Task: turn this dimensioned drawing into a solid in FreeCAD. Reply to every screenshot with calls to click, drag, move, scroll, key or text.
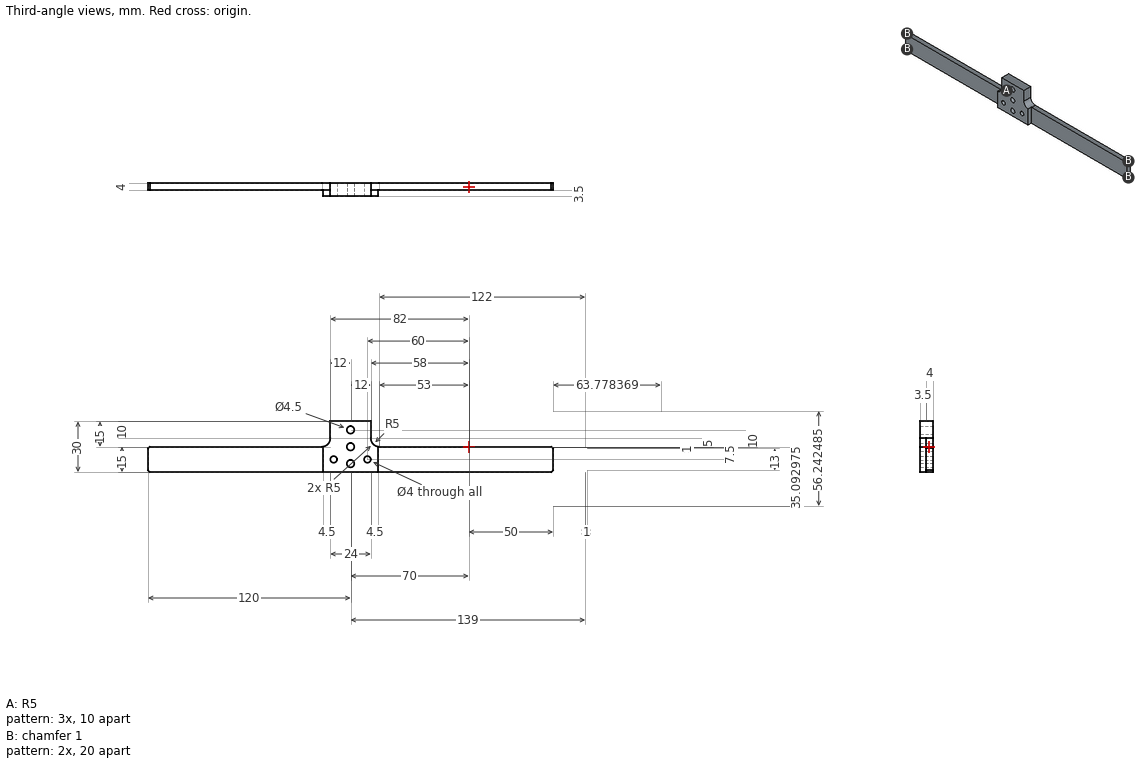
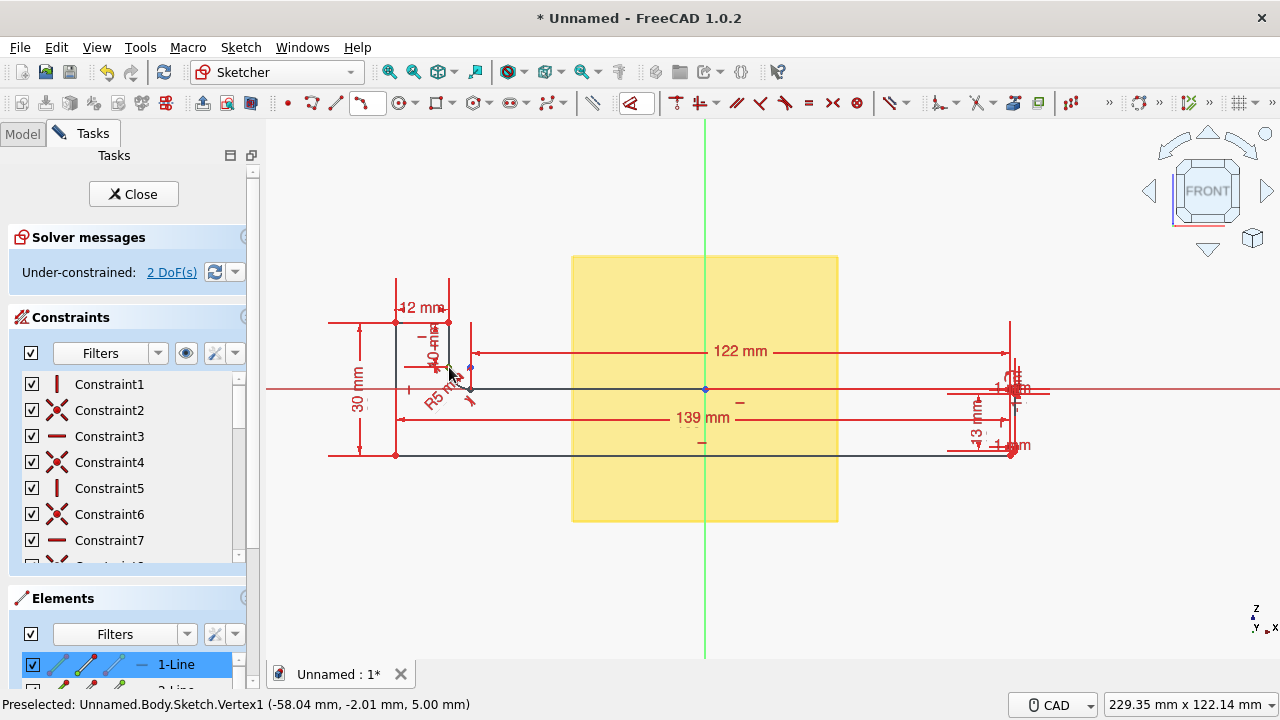
click(648, 104)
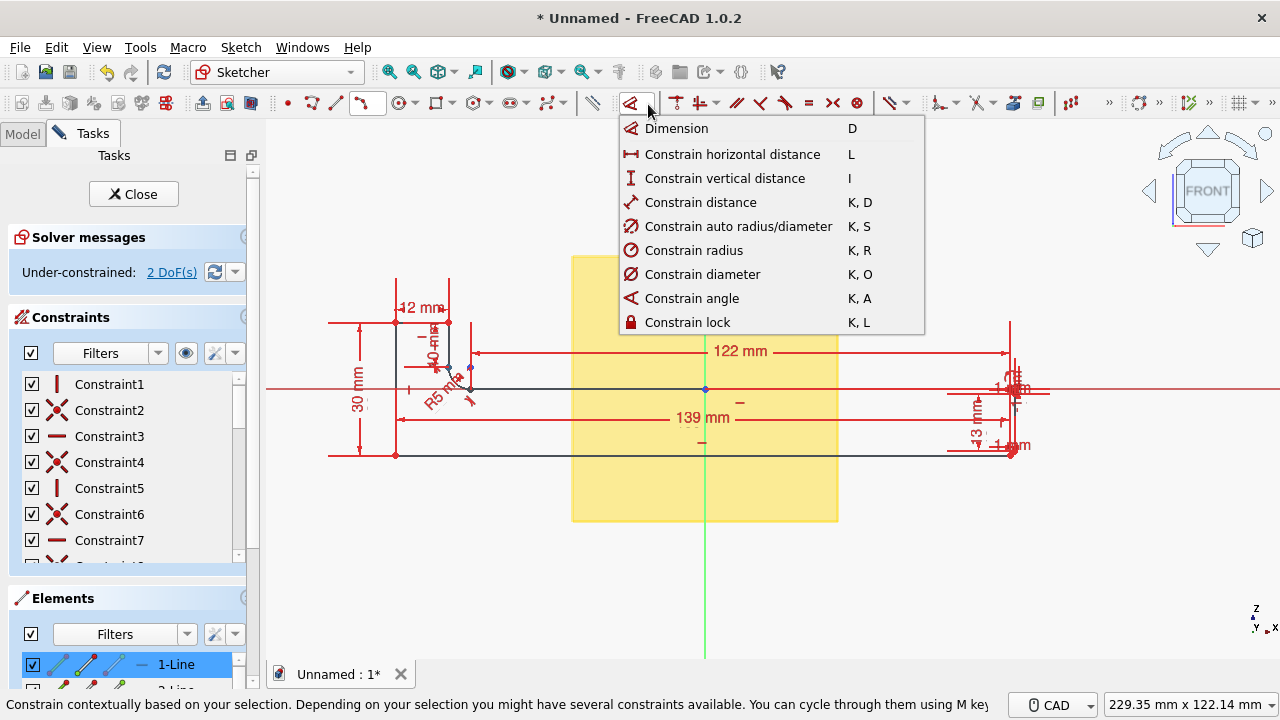
click(772, 154)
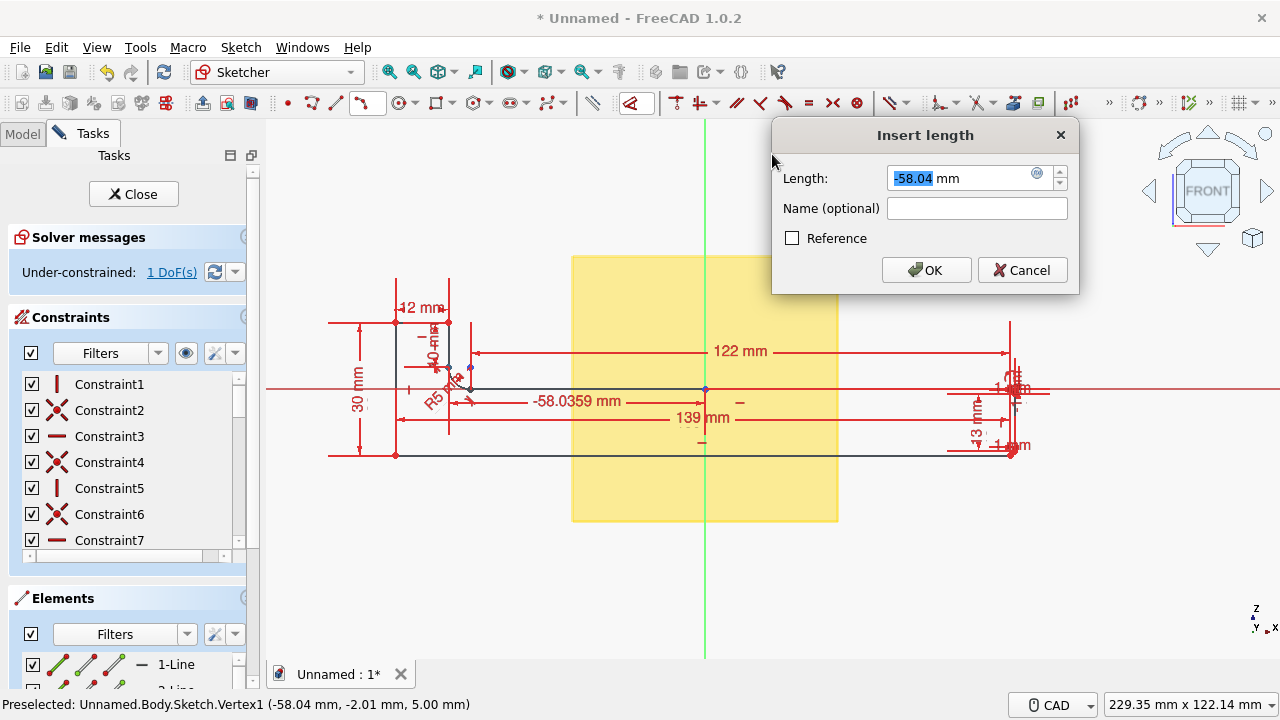
text(-58)
key(Return)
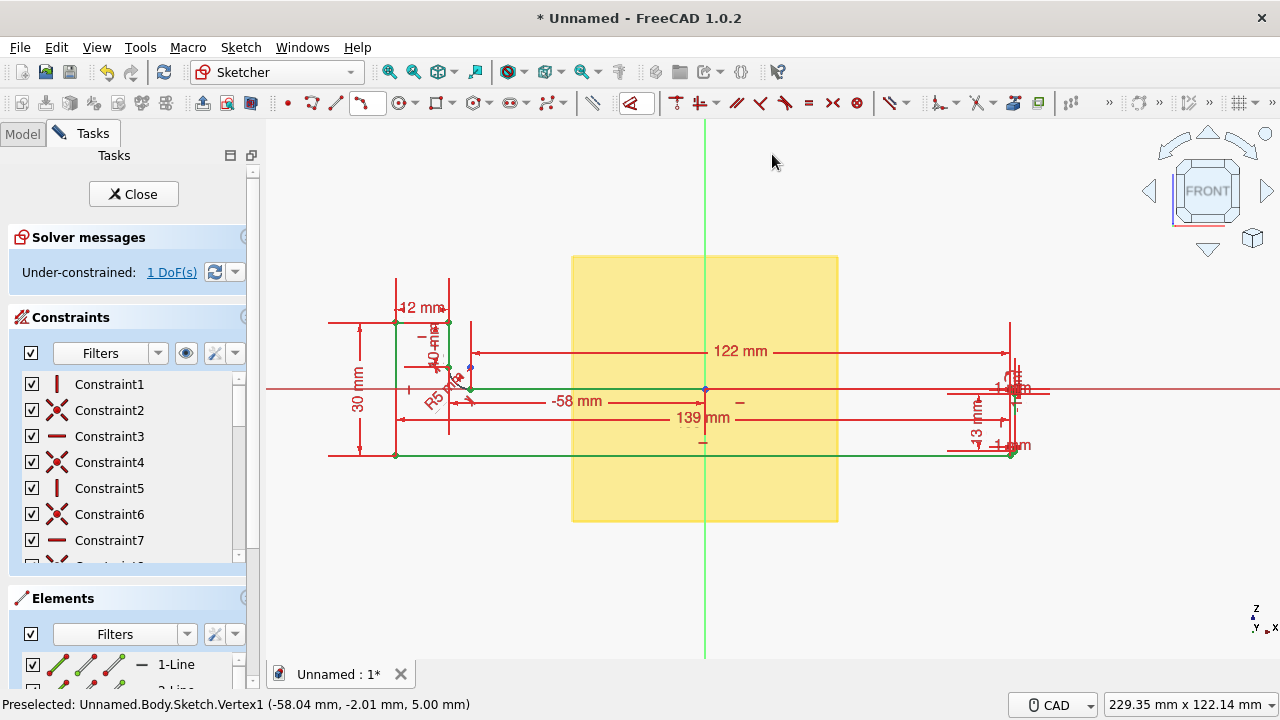
click(471, 389)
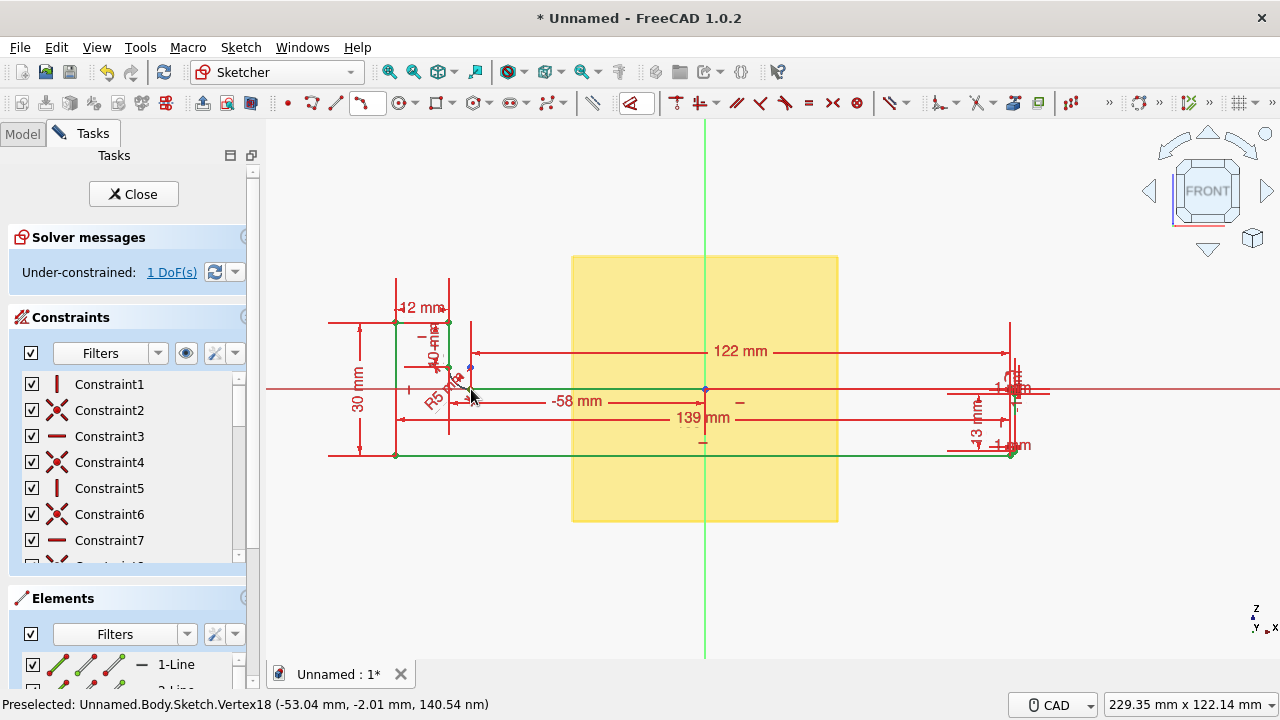
click(648, 104)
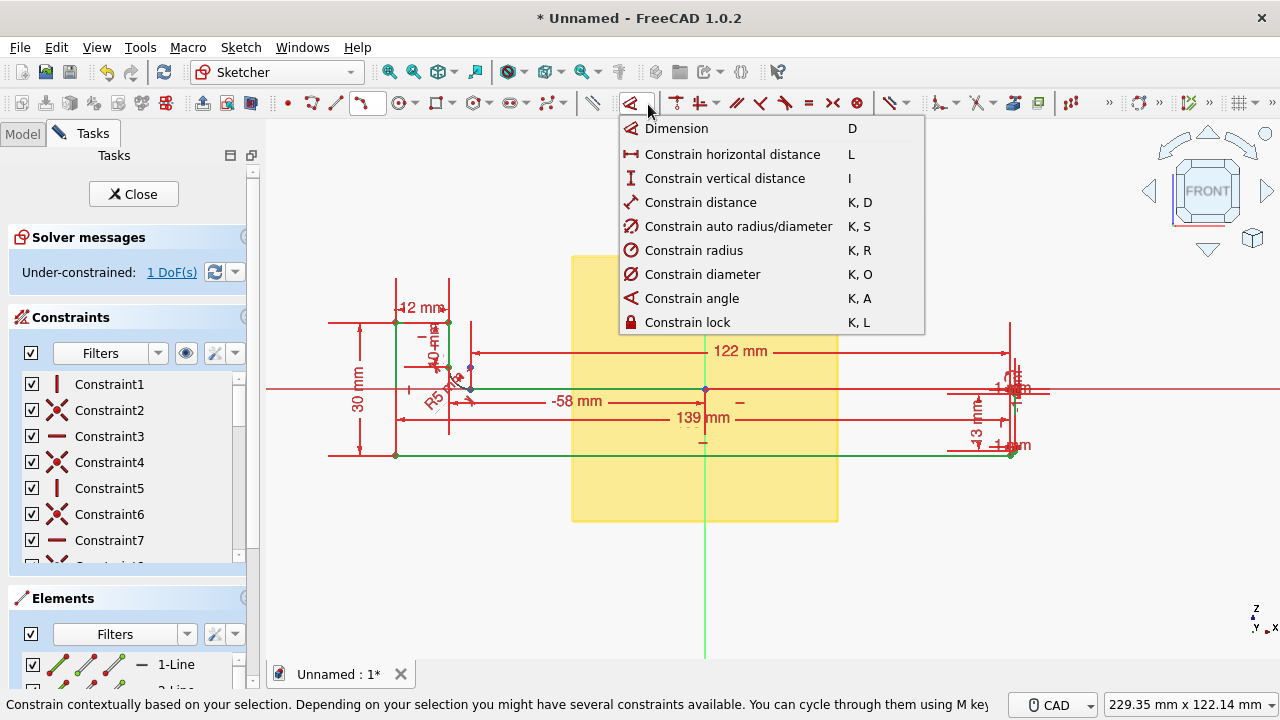
click(772, 154)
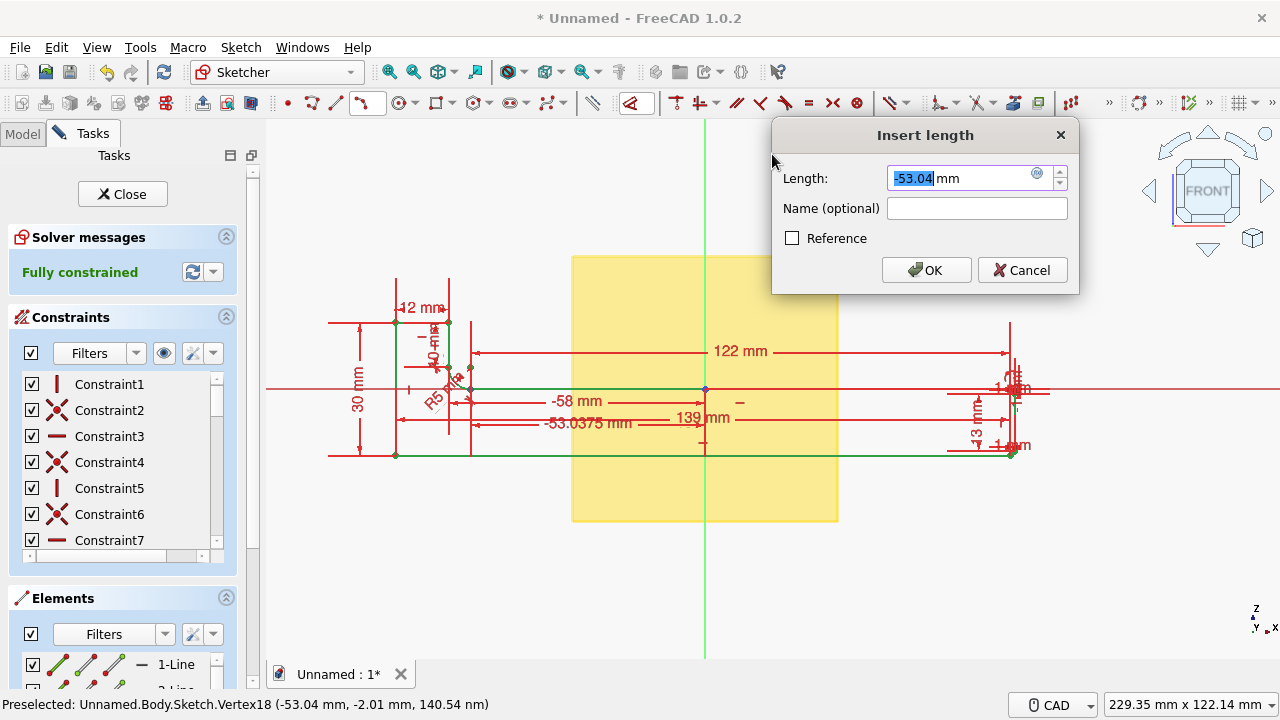
text(-53)
key(Return)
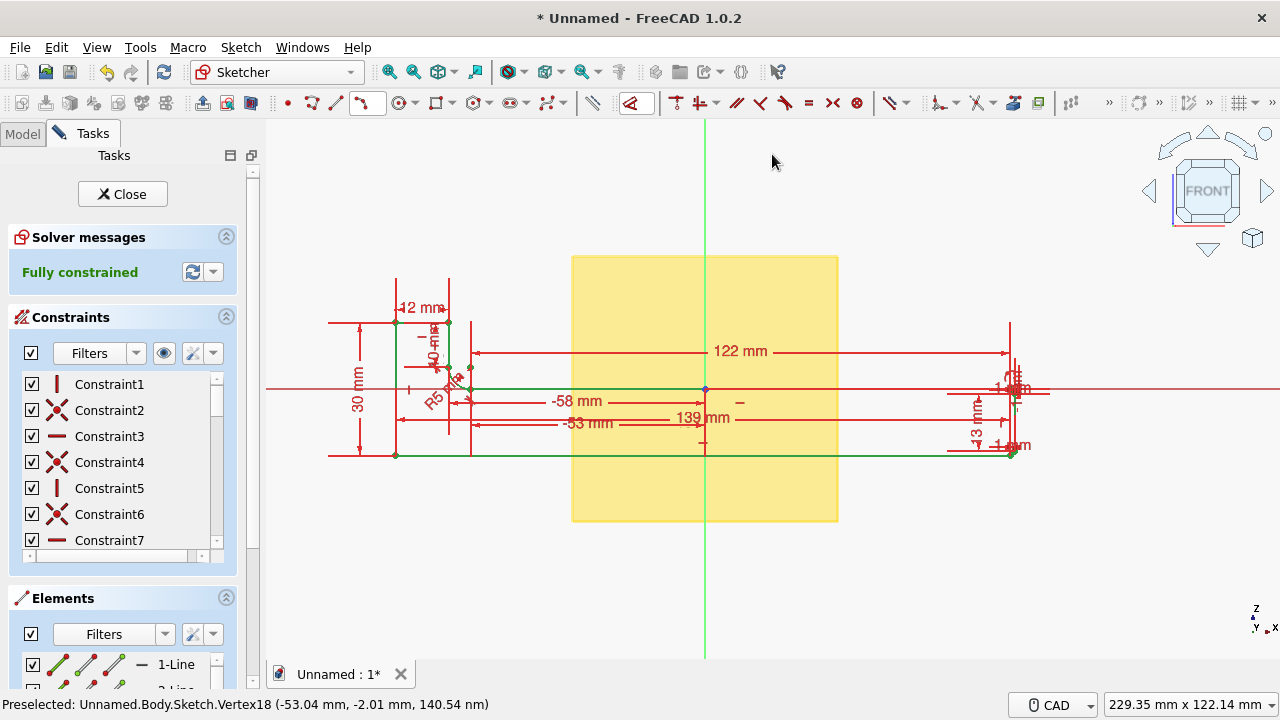
click(123, 194)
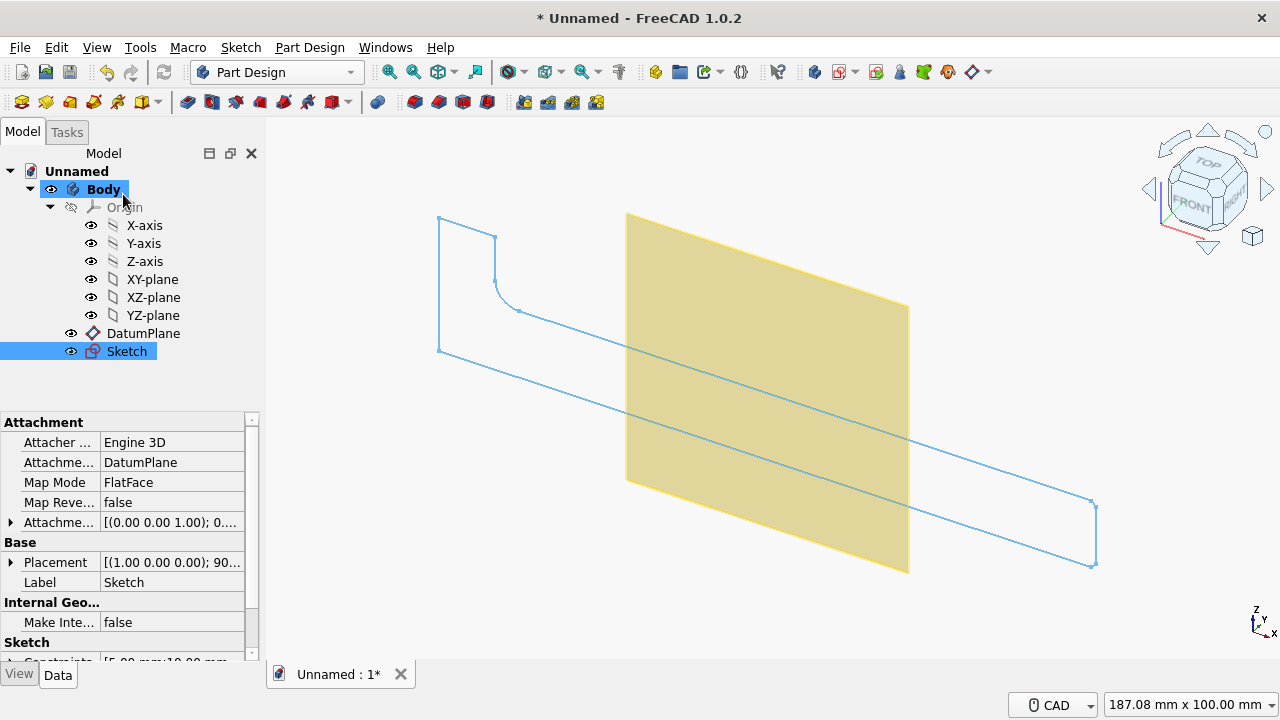
click(22, 102)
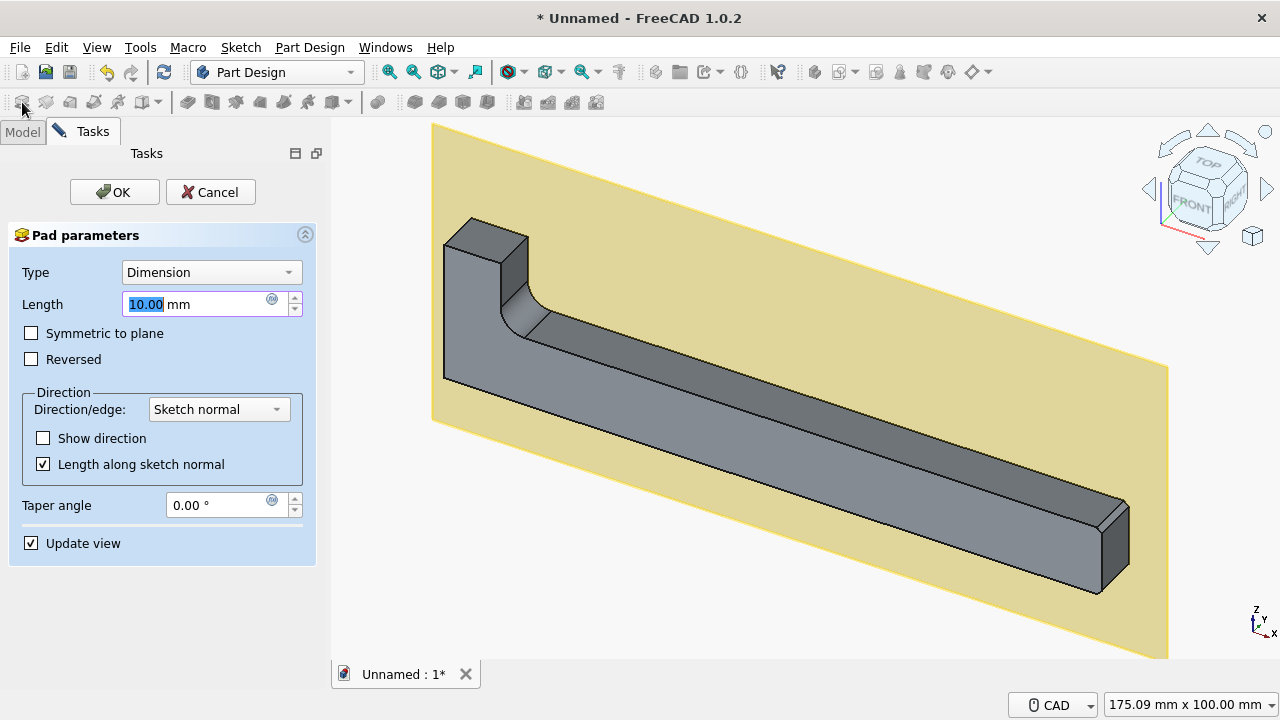
text(4)
key(Tab)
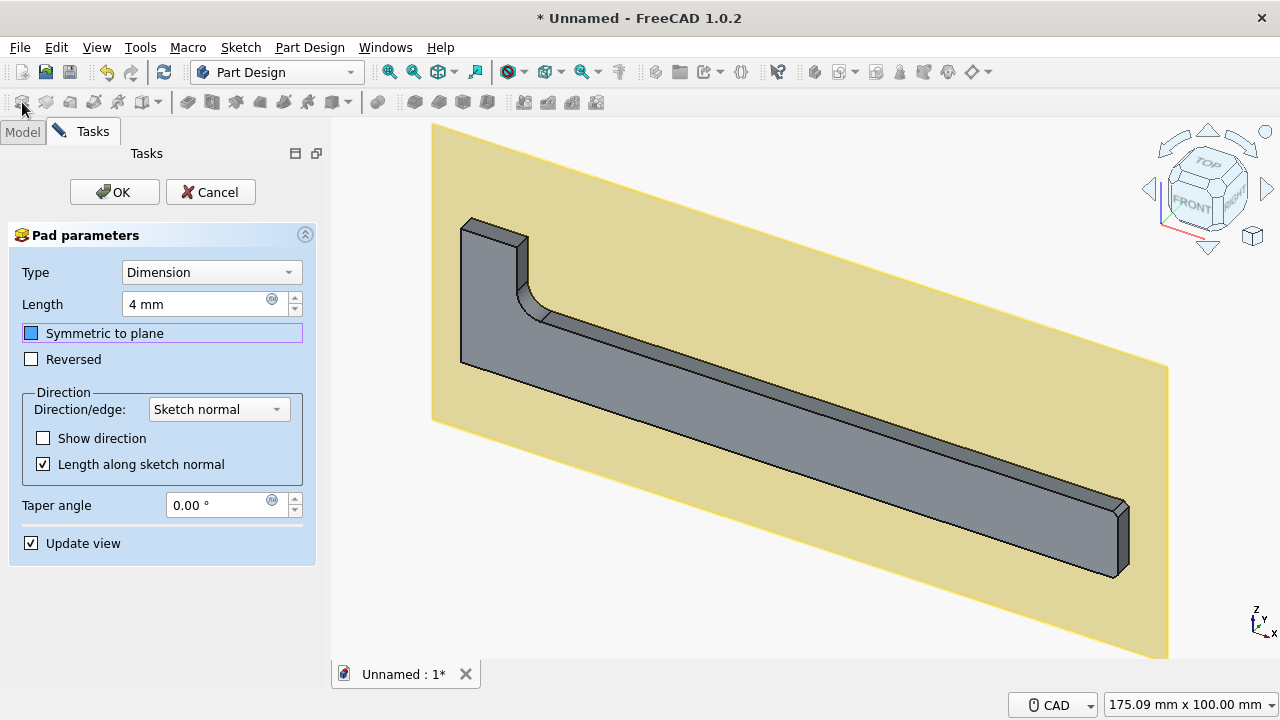
click(30, 359)